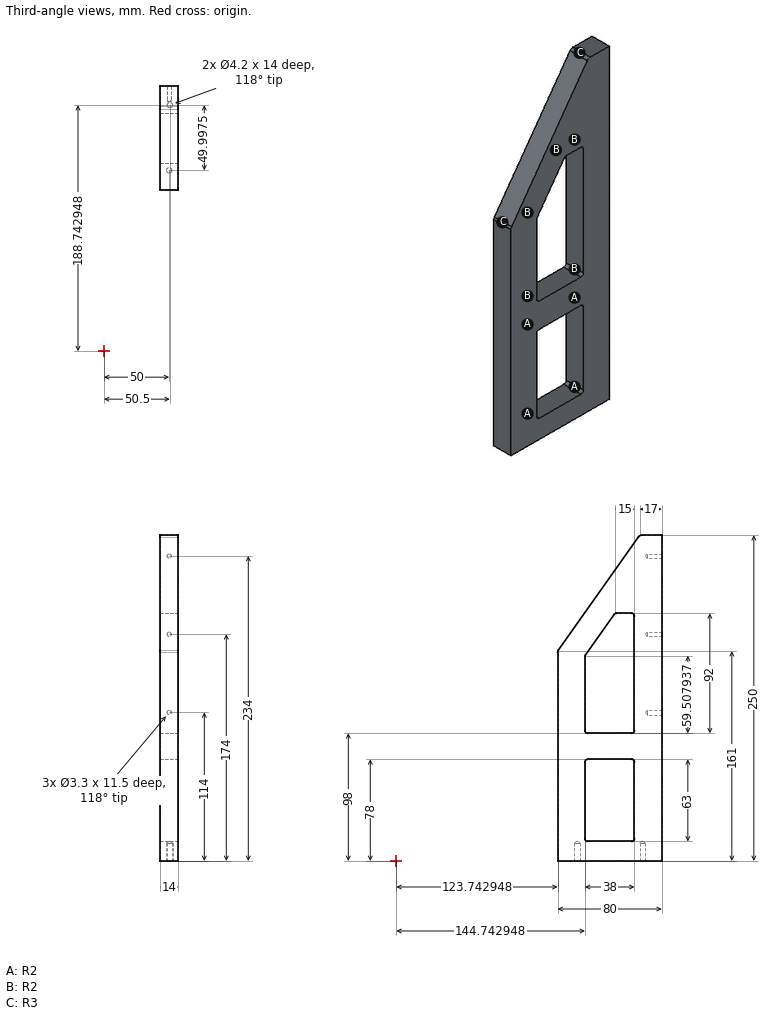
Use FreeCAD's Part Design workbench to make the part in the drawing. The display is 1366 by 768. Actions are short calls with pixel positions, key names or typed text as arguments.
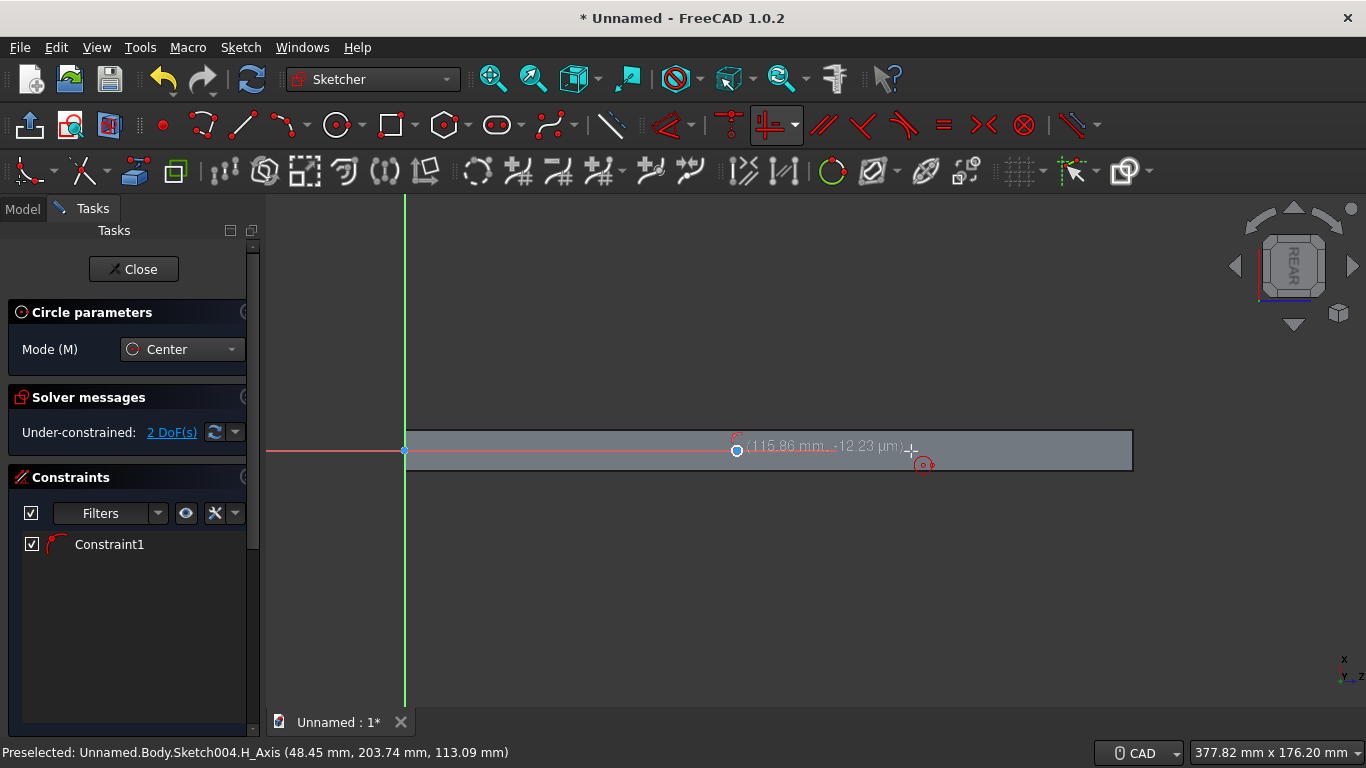
click(911, 451)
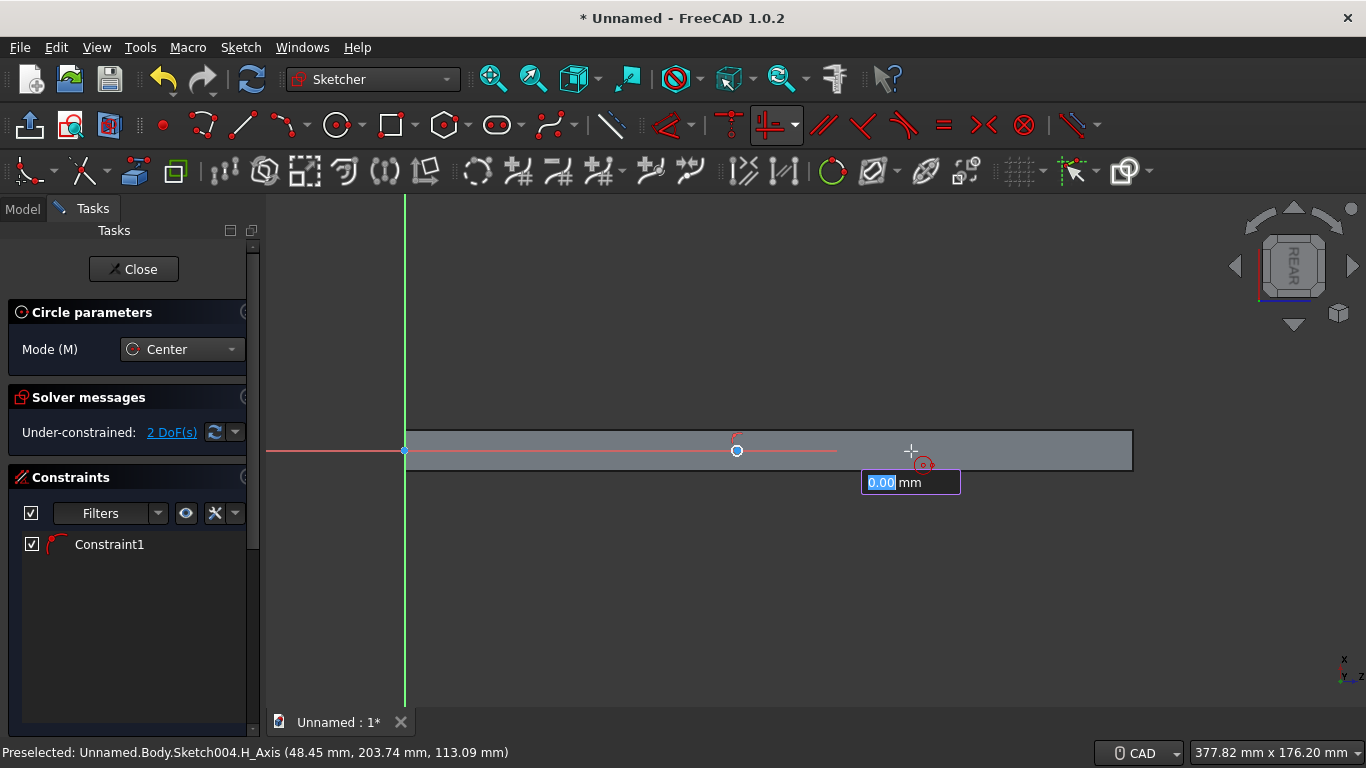
scroll(910, 455, up, 7)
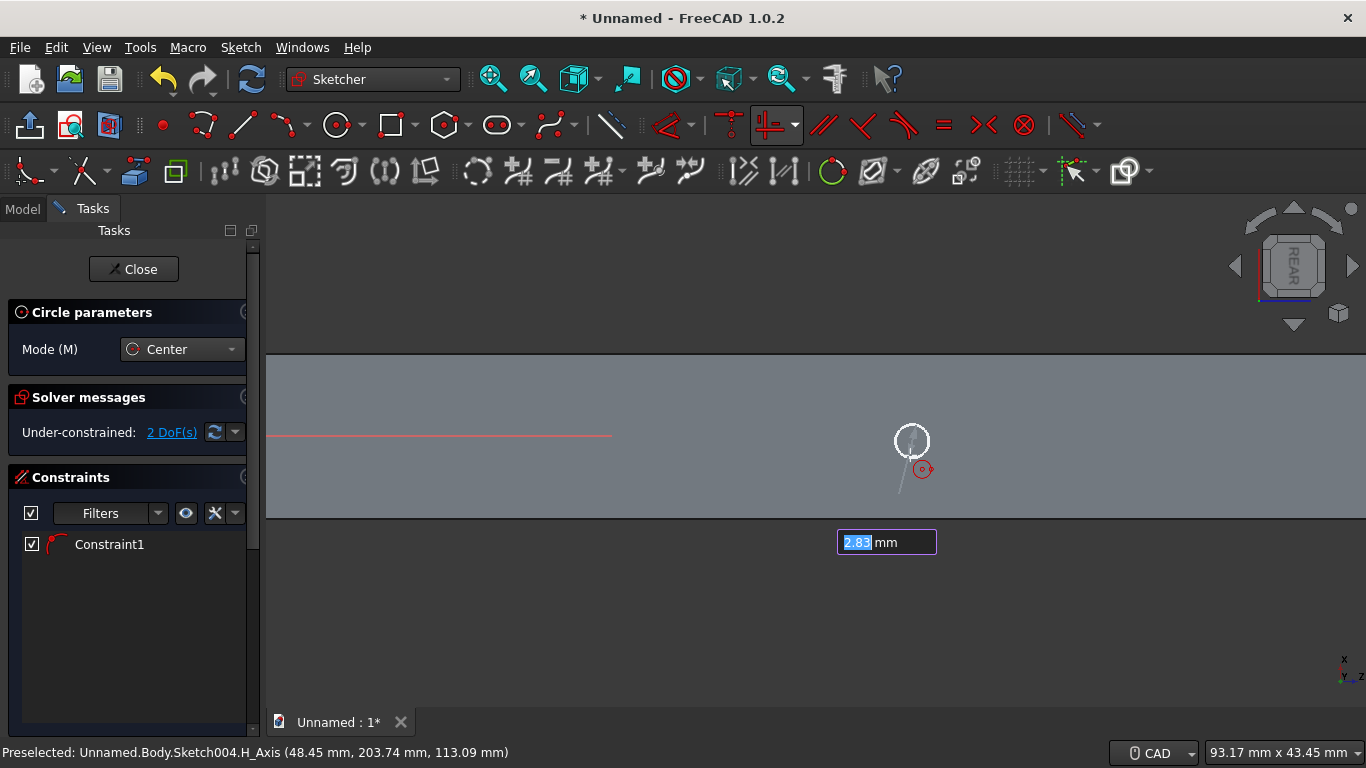
click(907, 455)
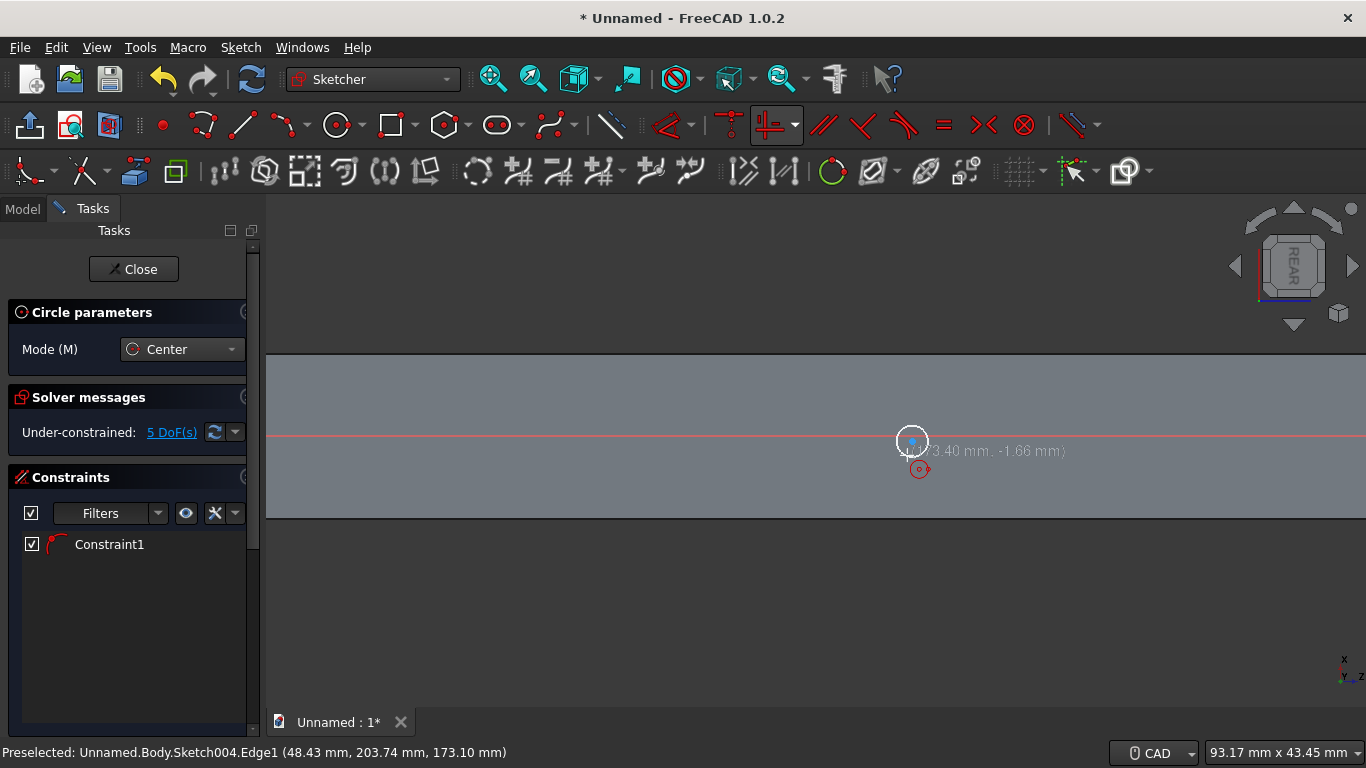
scroll(910, 455, down, 7)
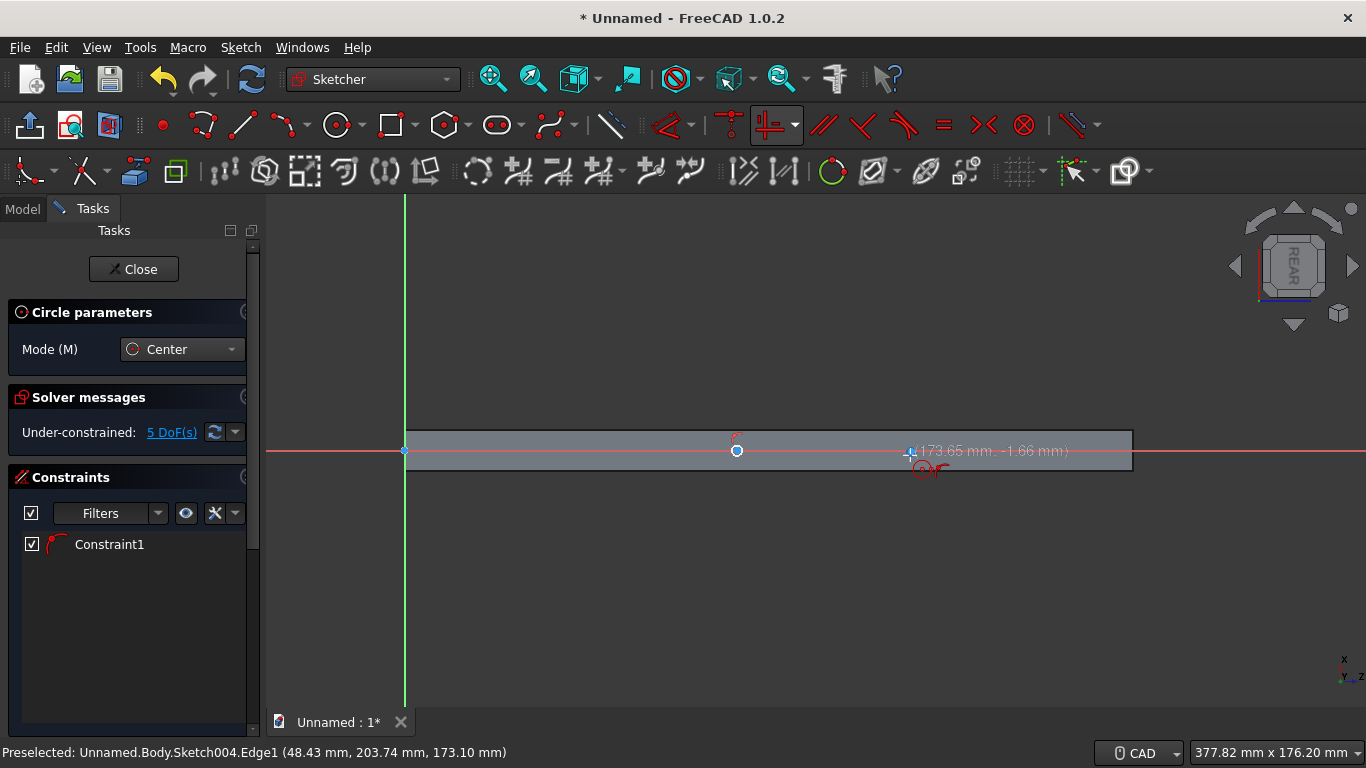
scroll(1086, 451, up, 8)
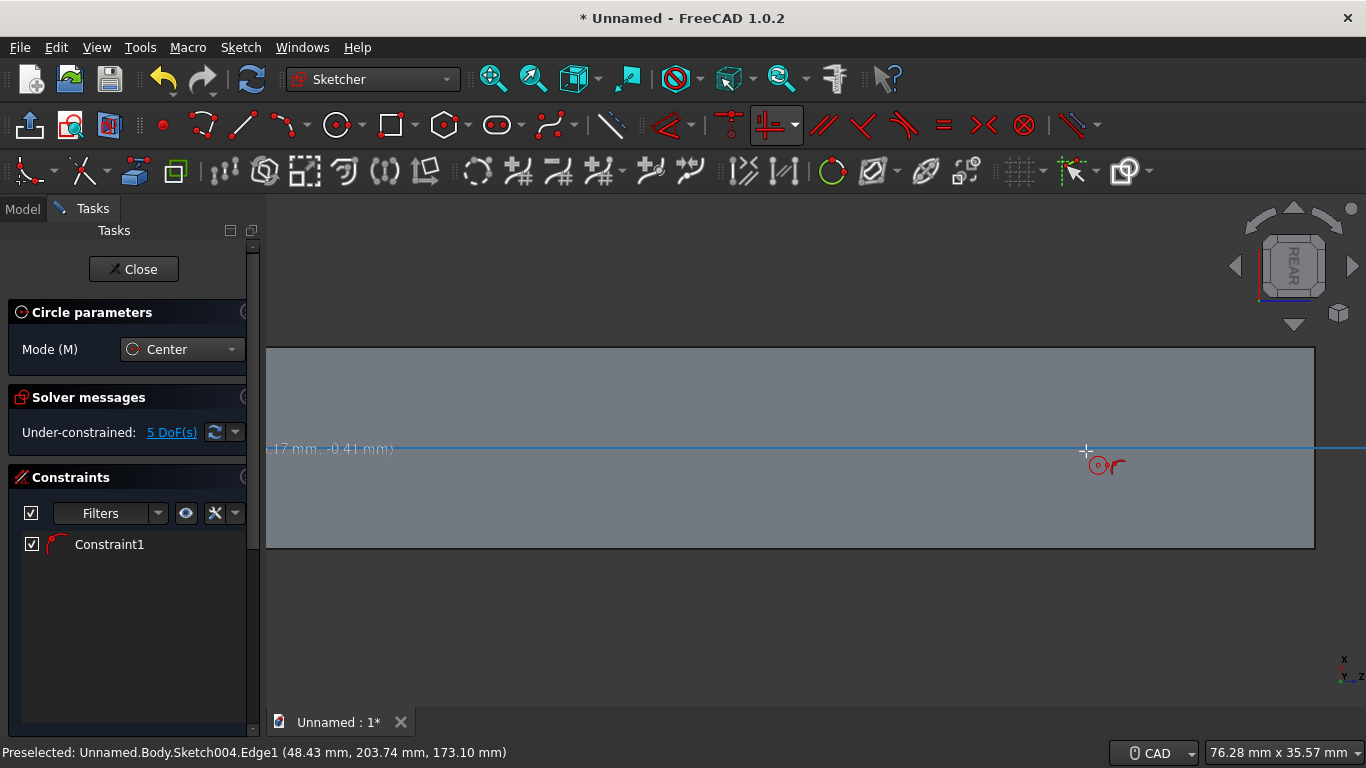
scroll(1086, 451, down, 8)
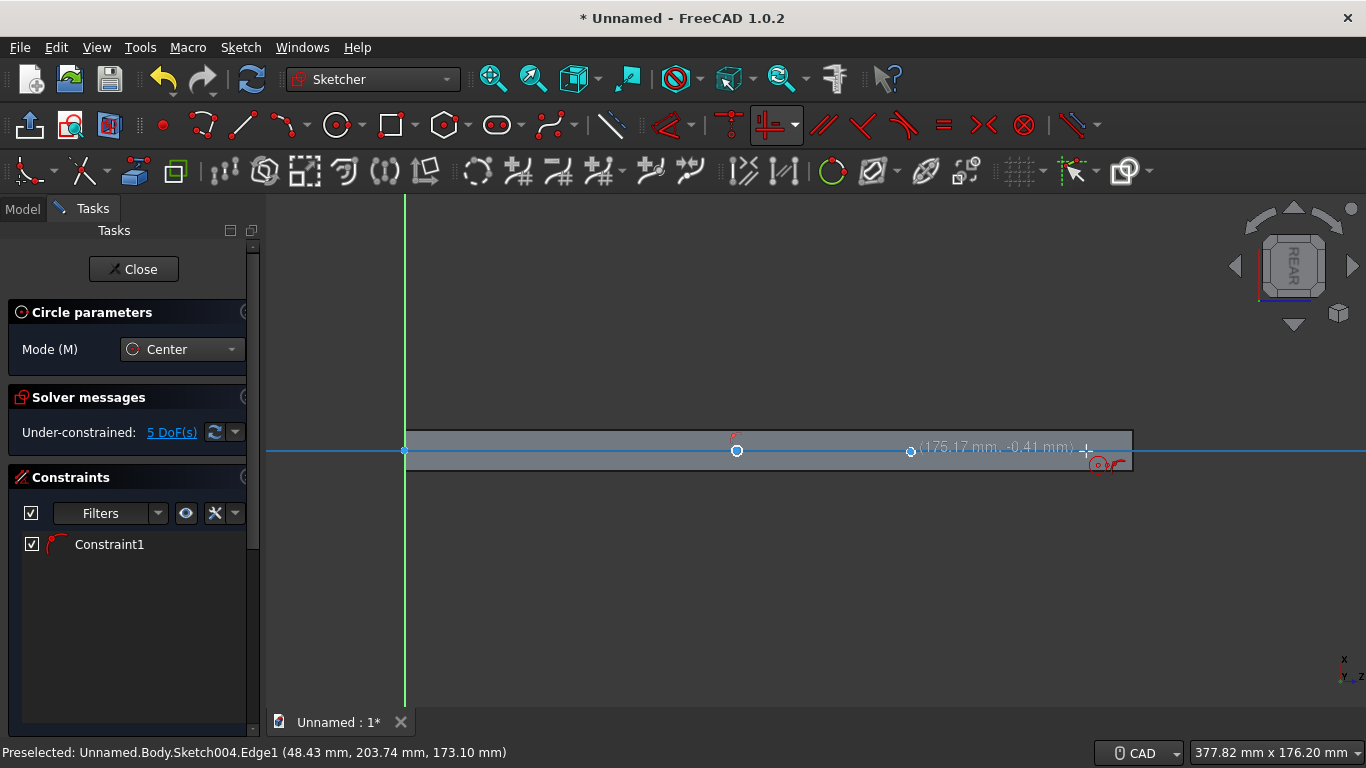
click(1086, 451)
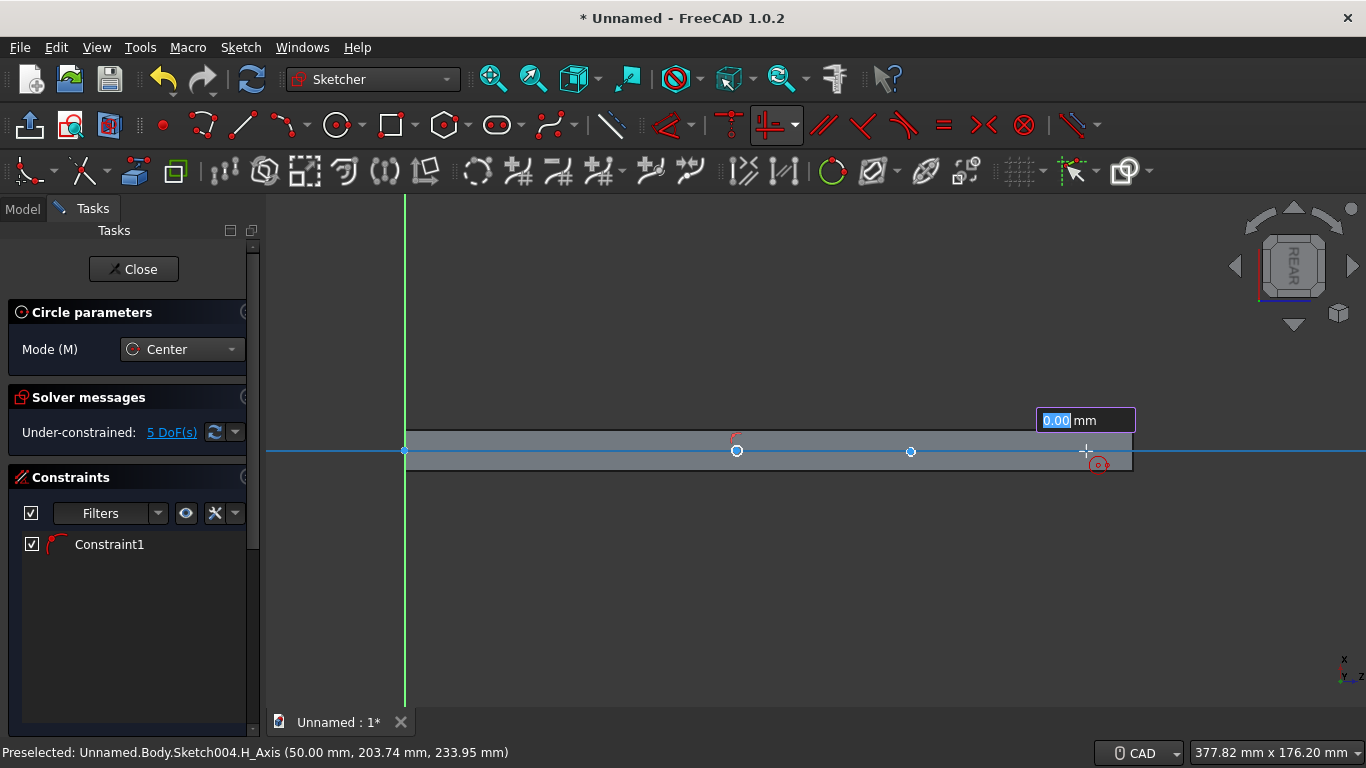
scroll(1085, 455, up, 7)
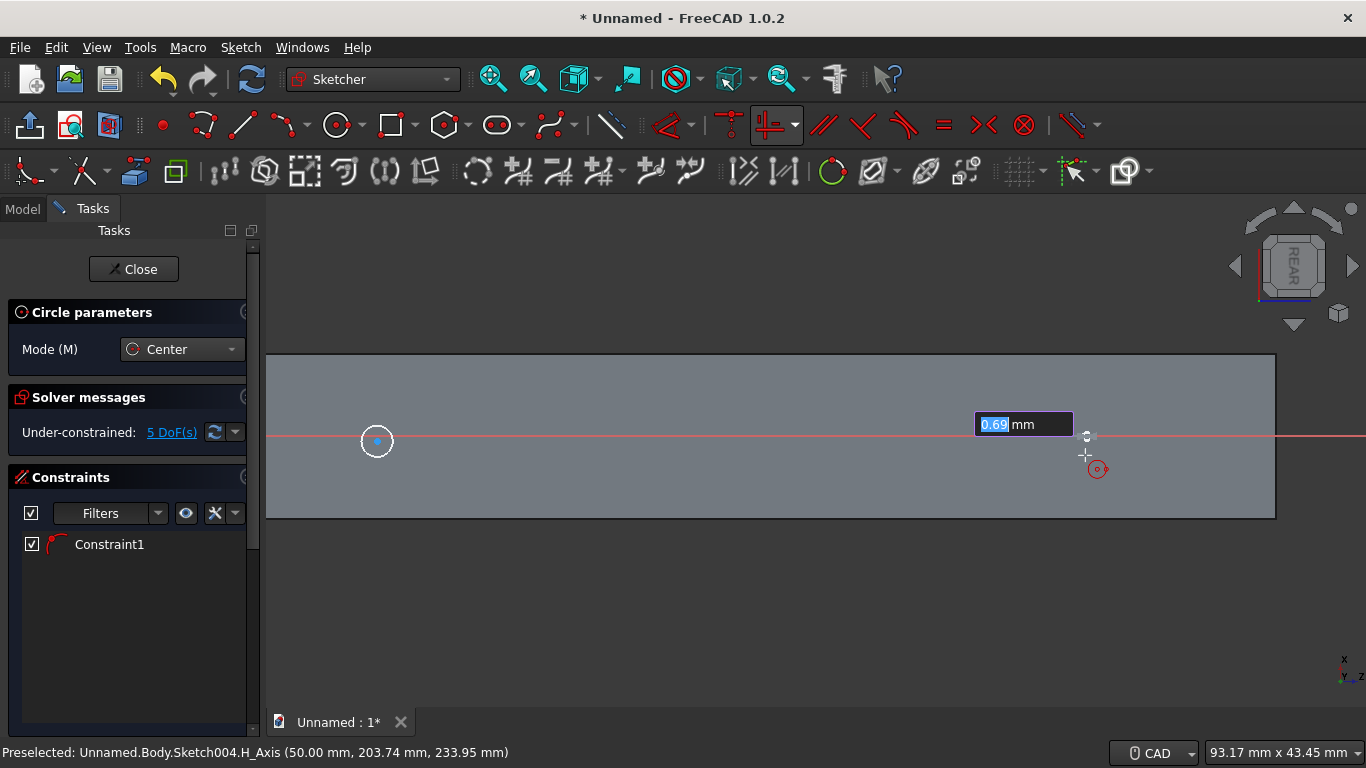
click(1081, 455)
key(Escape)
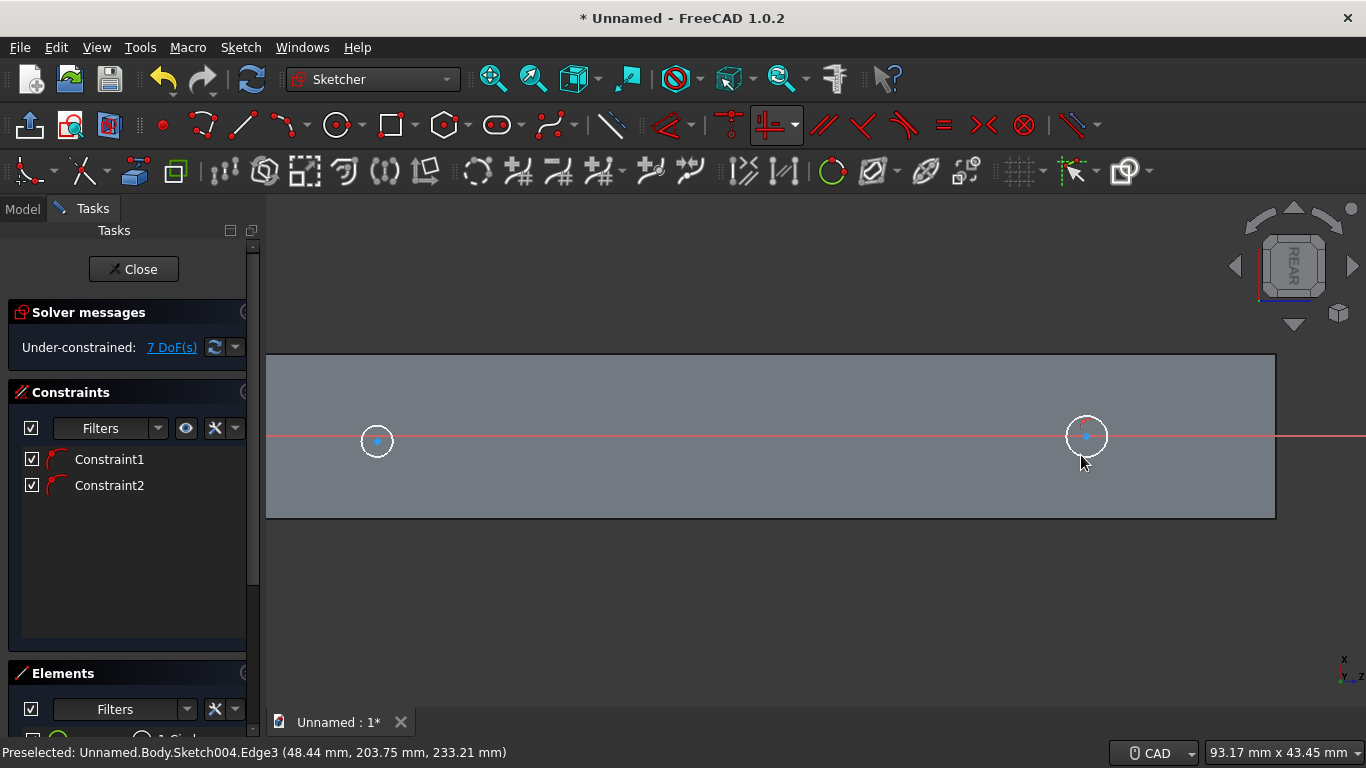
scroll(1085, 455, down, 7)